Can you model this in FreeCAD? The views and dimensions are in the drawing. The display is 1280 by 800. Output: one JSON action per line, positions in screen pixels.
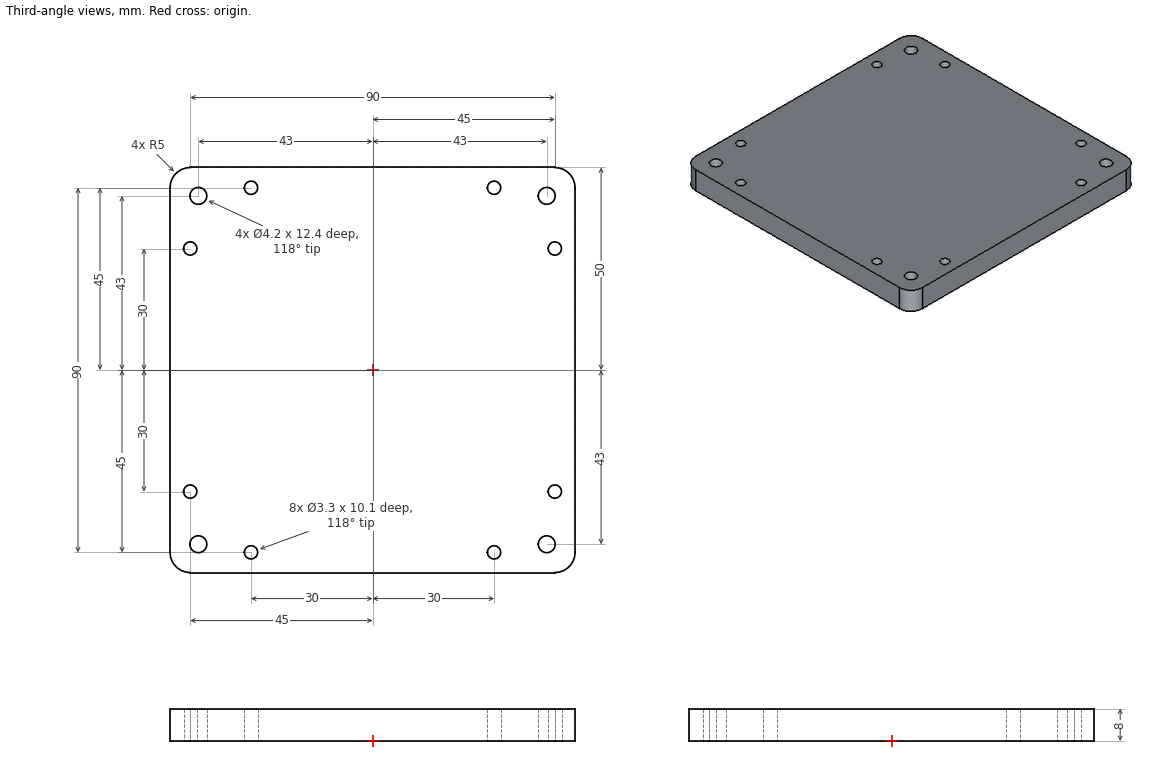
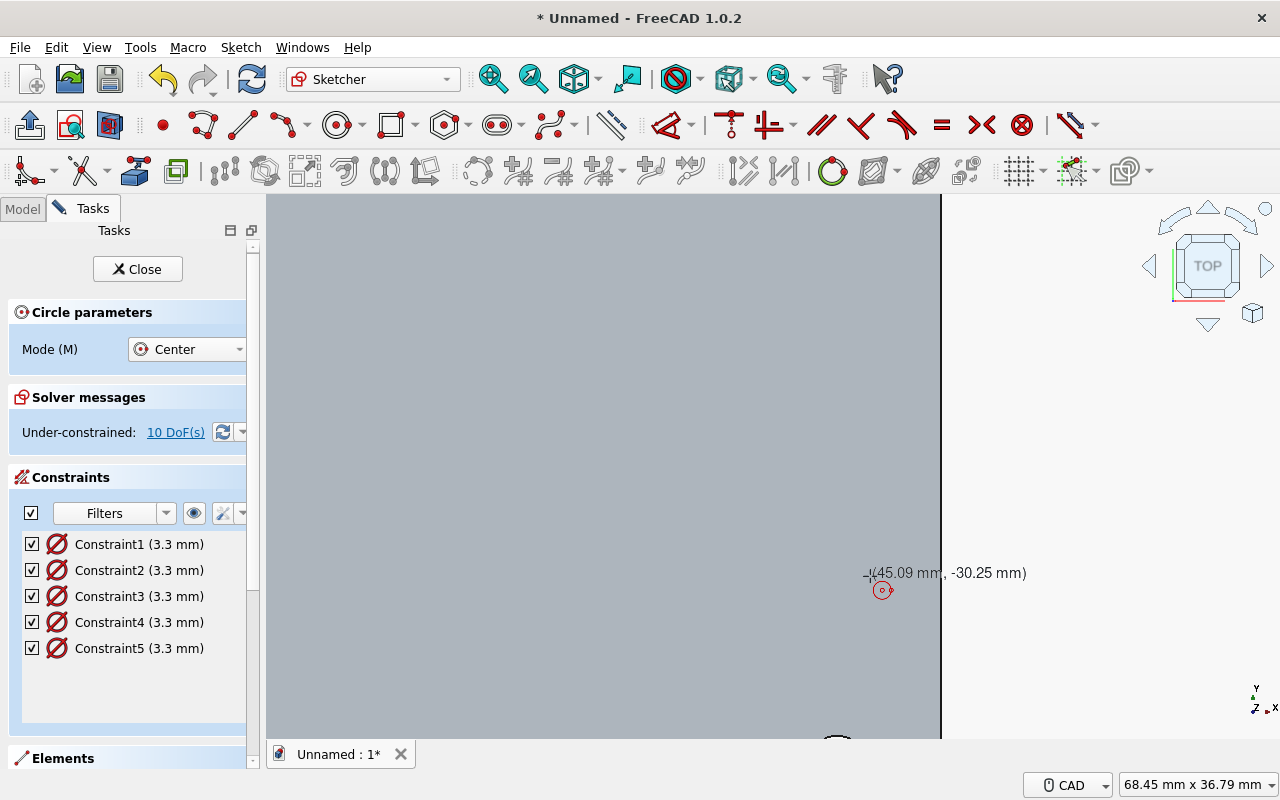
{"action": "scroll", "coordinate": [870, 577], "scroll_direction": "down", "scroll_amount": 7}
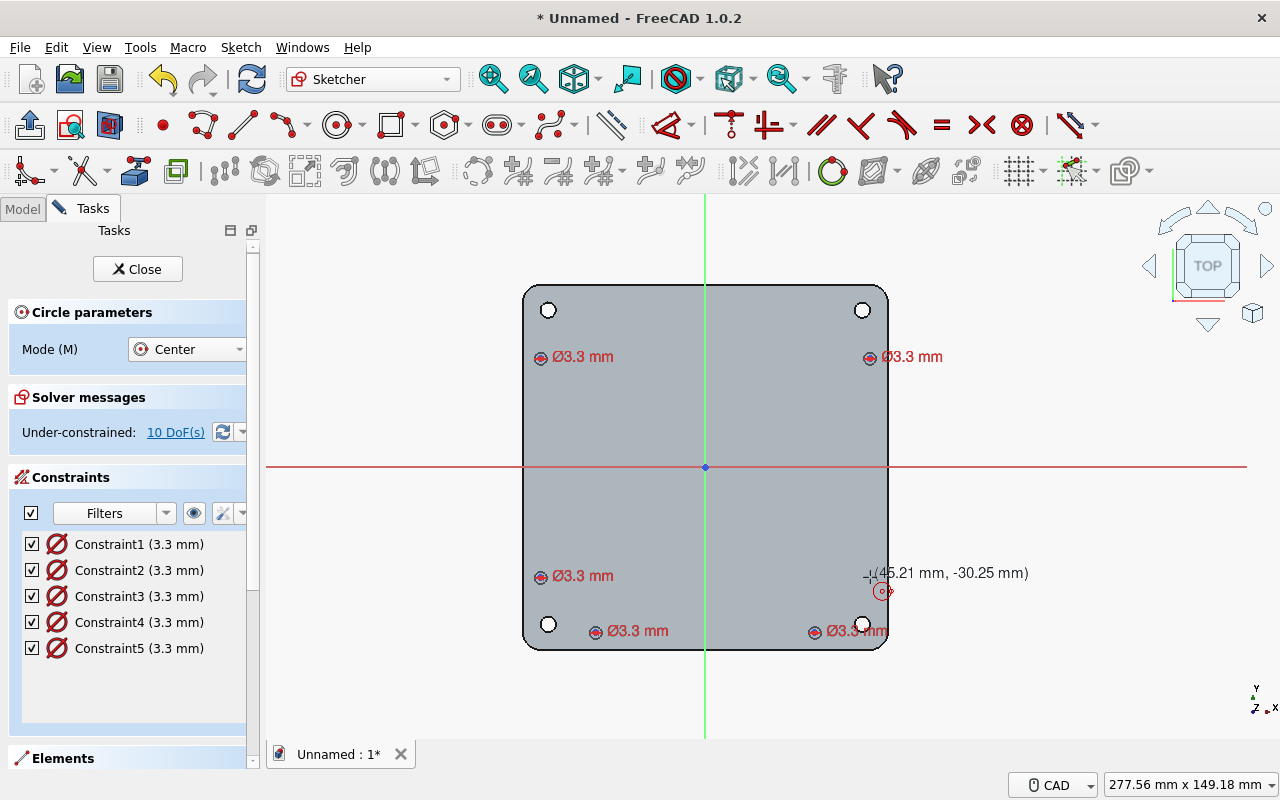
{"action": "left_click", "coordinate": [870, 577]}
{"action": "mouse_move", "coordinate": [874, 573]}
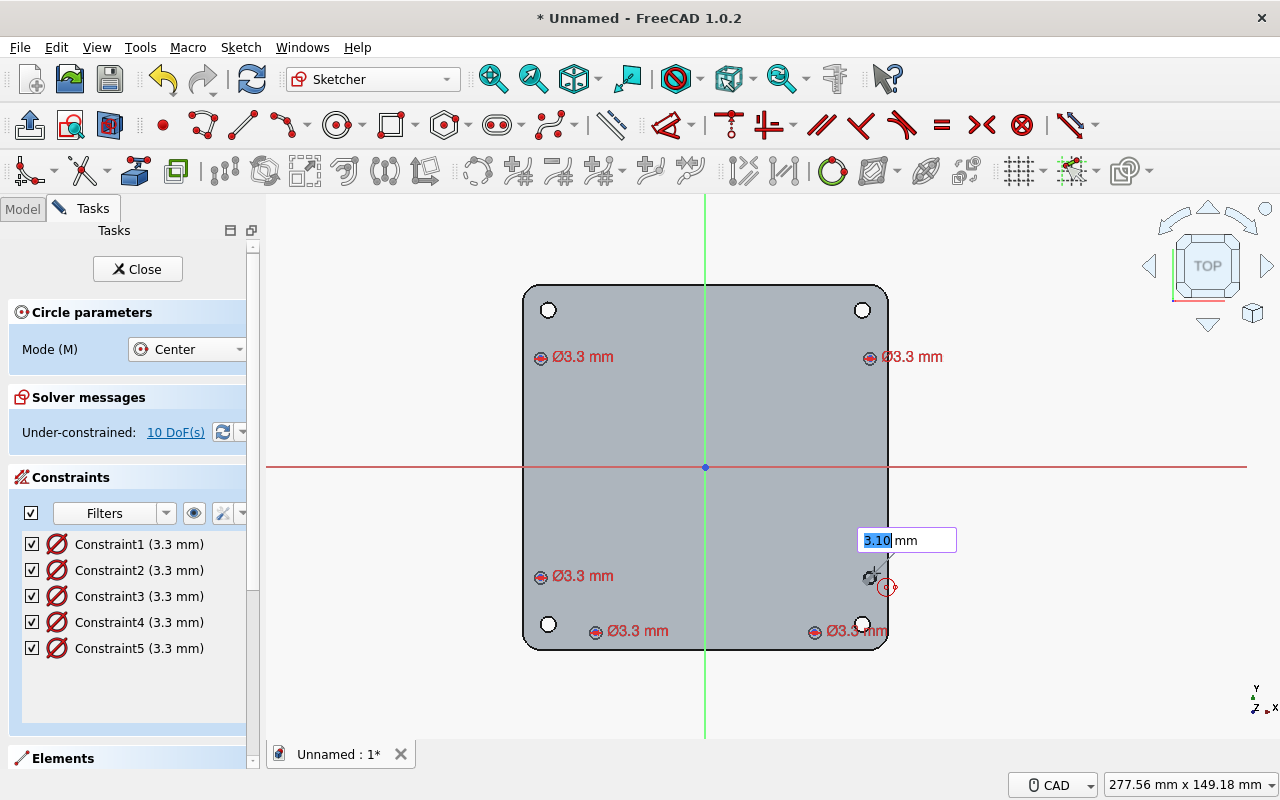
{"action": "type", "text": "3.3"}
{"action": "key", "text": "Return"}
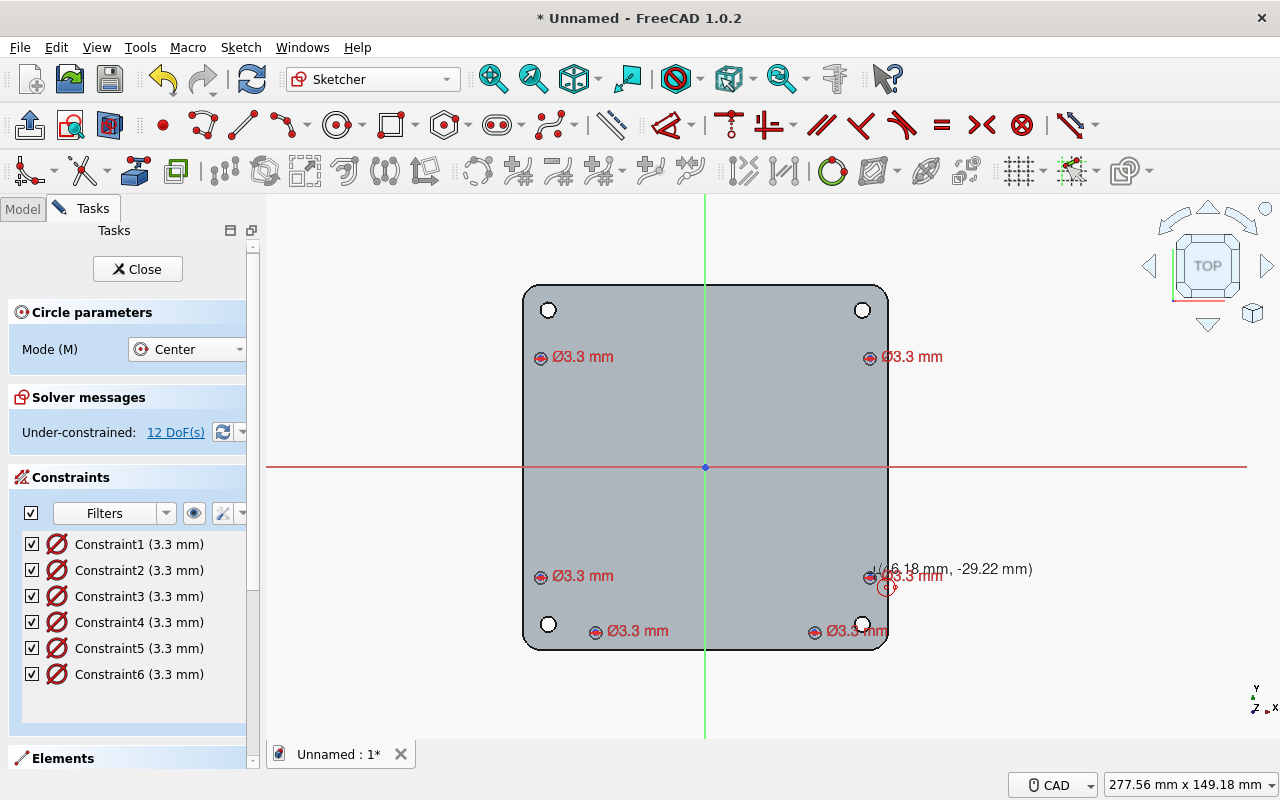
{"action": "scroll", "coordinate": [596, 303], "scroll_direction": "up", "scroll_amount": 7}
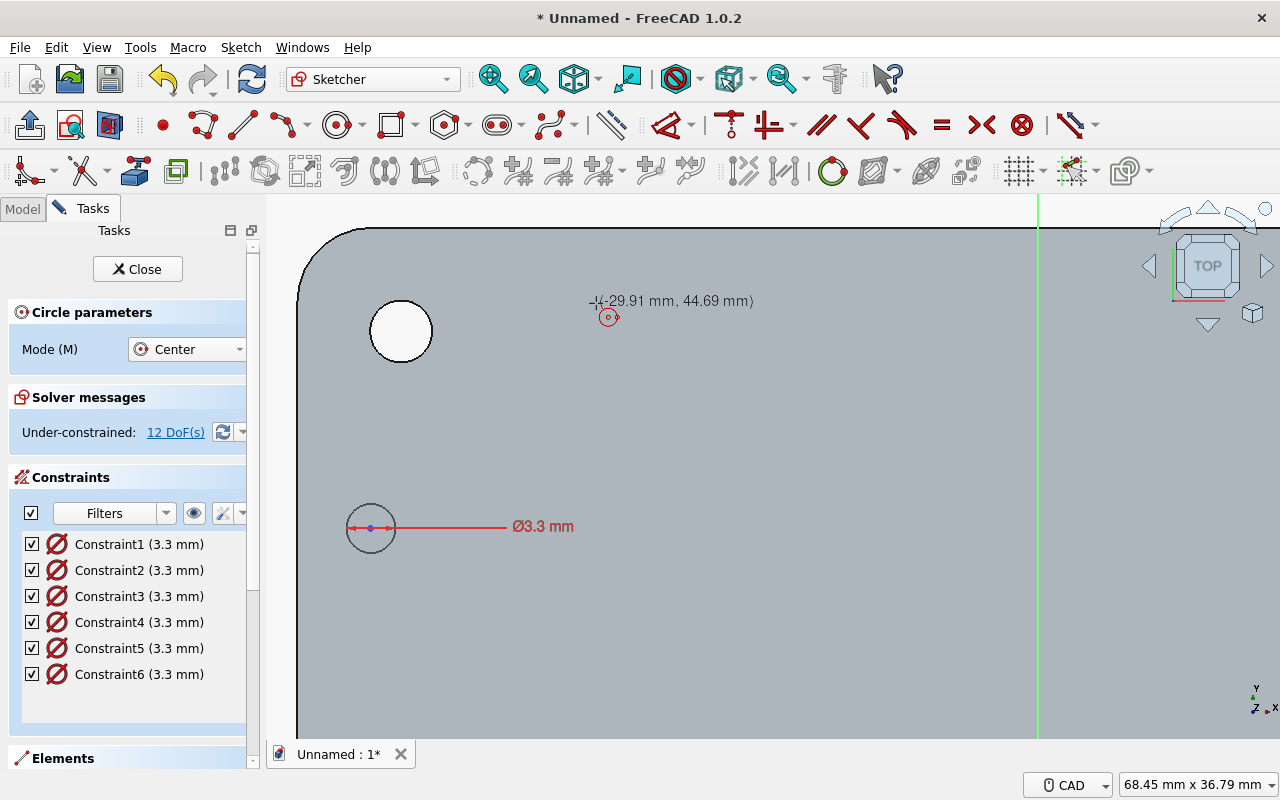
{"action": "scroll", "coordinate": [595, 302], "scroll_direction": "down", "scroll_amount": 7}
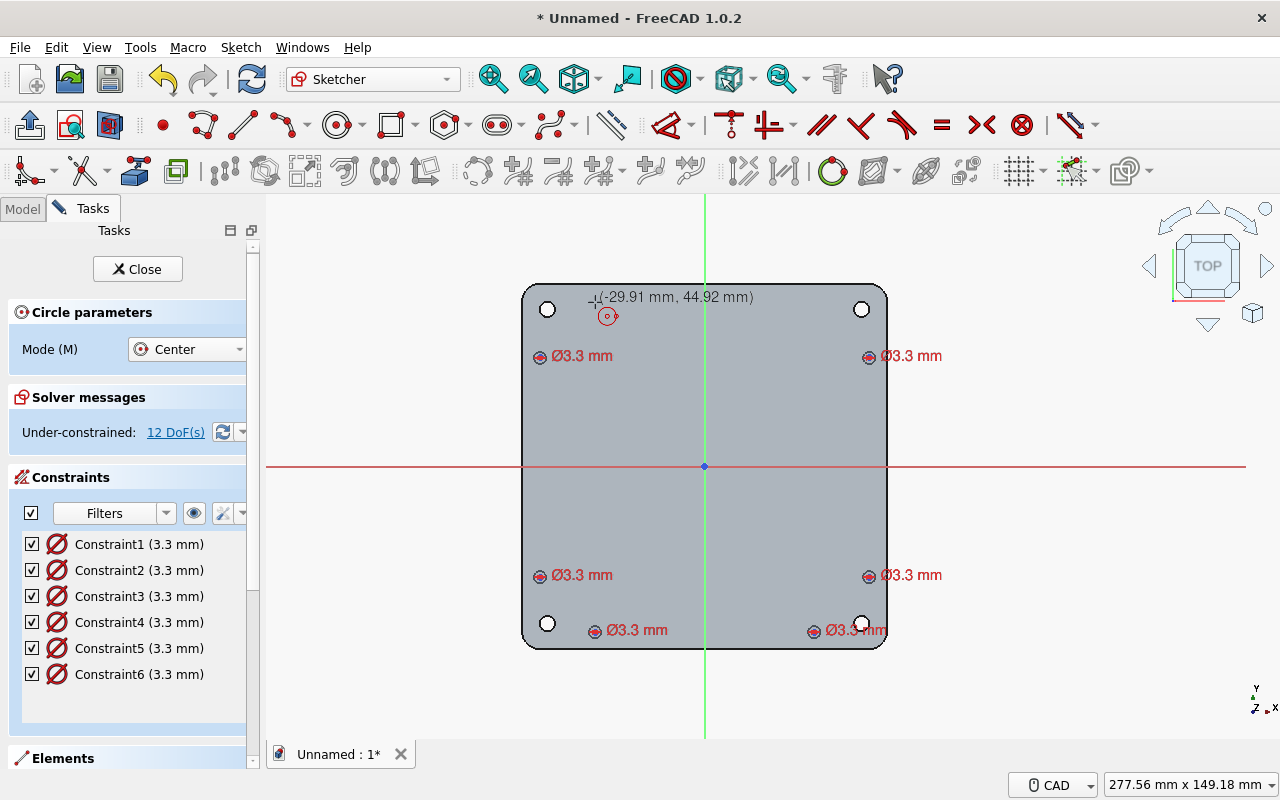
{"action": "left_click", "coordinate": [595, 302]}
{"action": "mouse_move", "coordinate": [599, 298]}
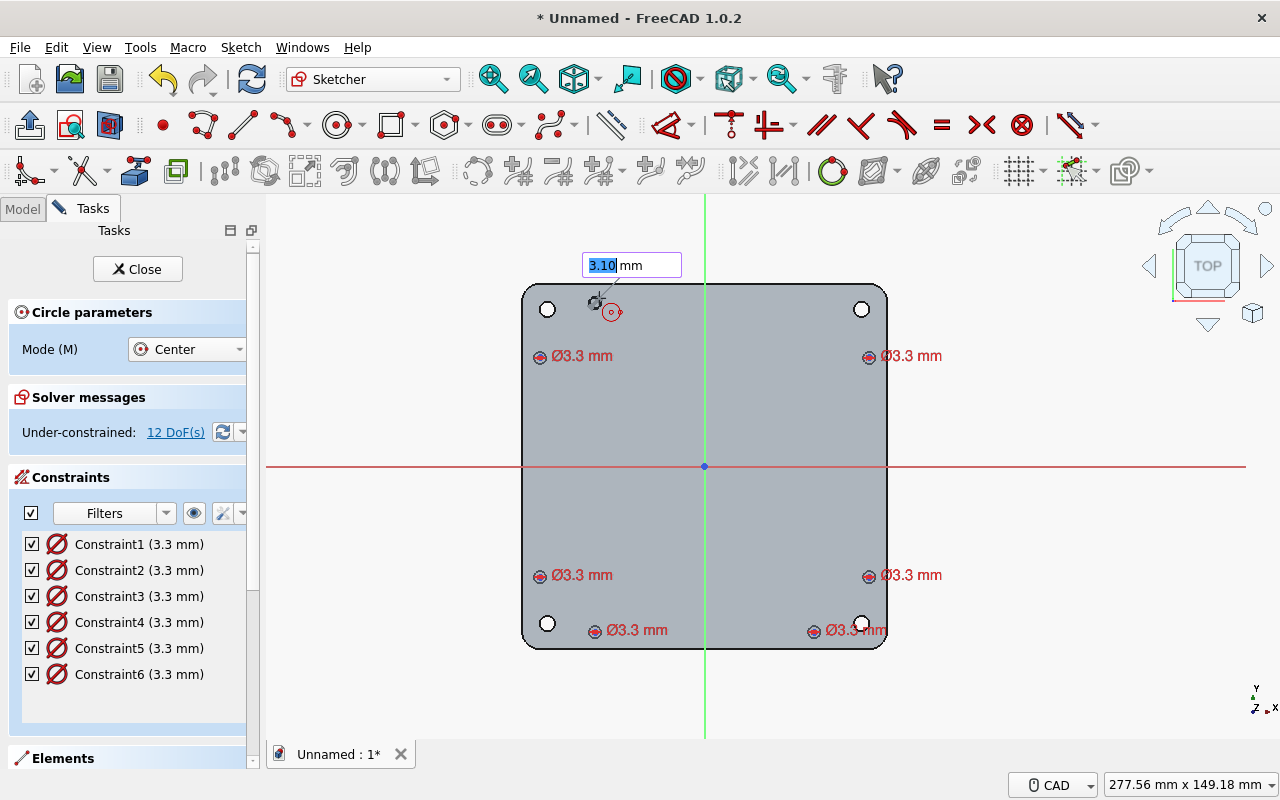
{"action": "type", "text": "3.3"}
{"action": "key", "text": "Return"}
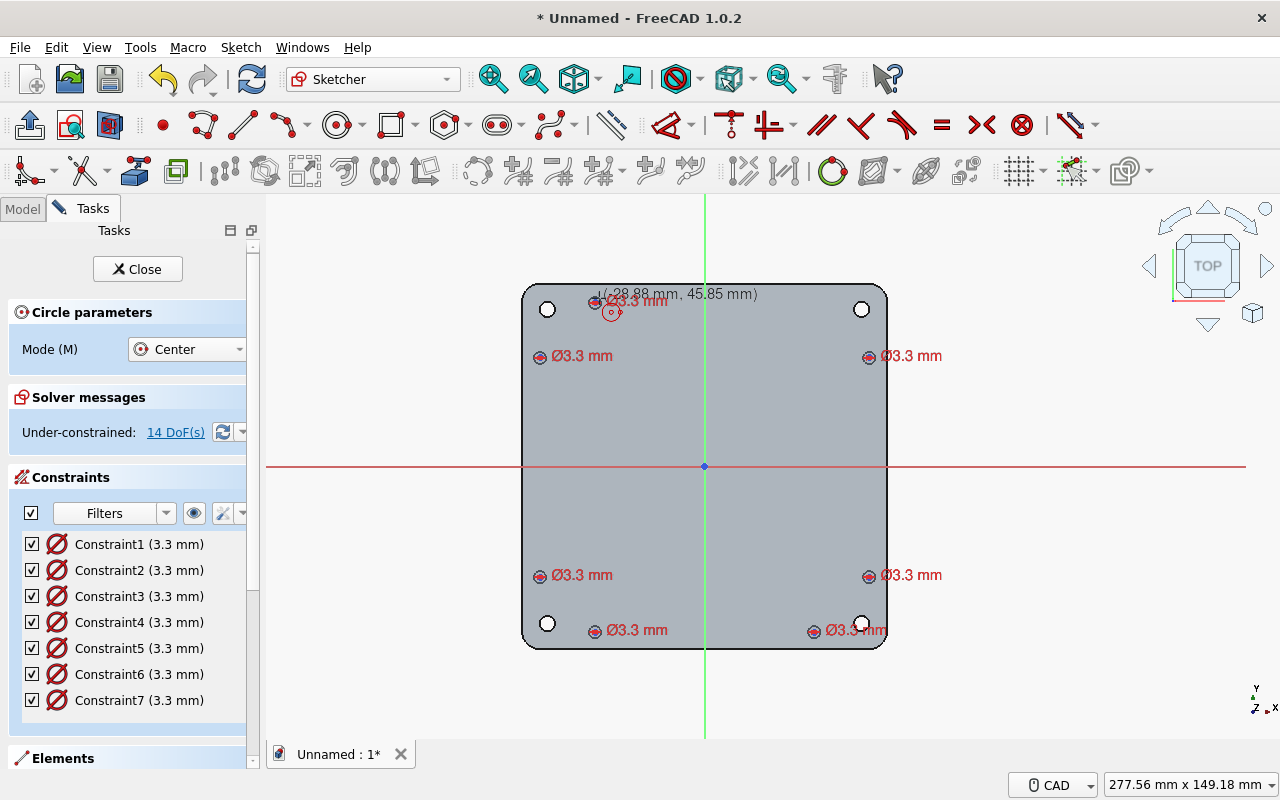
{"action": "scroll", "coordinate": [814, 302], "scroll_direction": "up", "scroll_amount": 7}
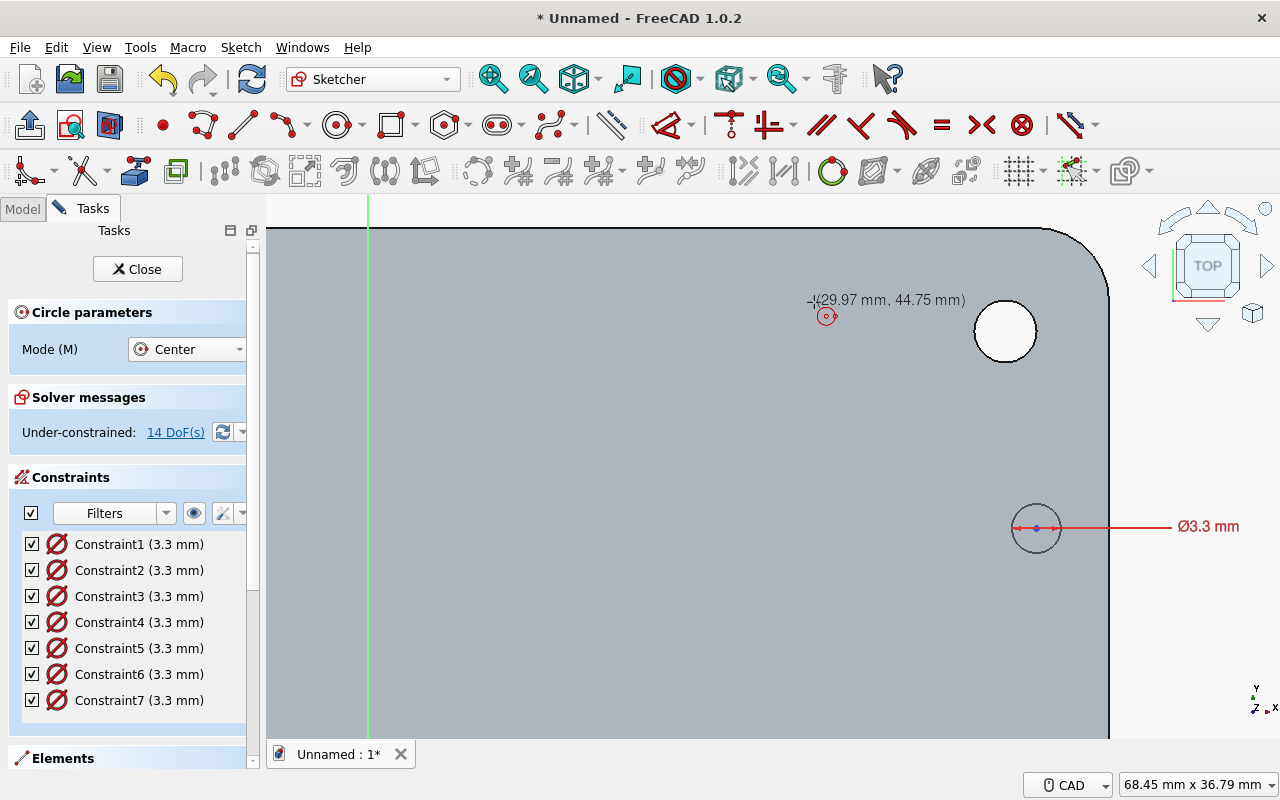
{"action": "scroll", "coordinate": [815, 302], "scroll_direction": "down", "scroll_amount": 7}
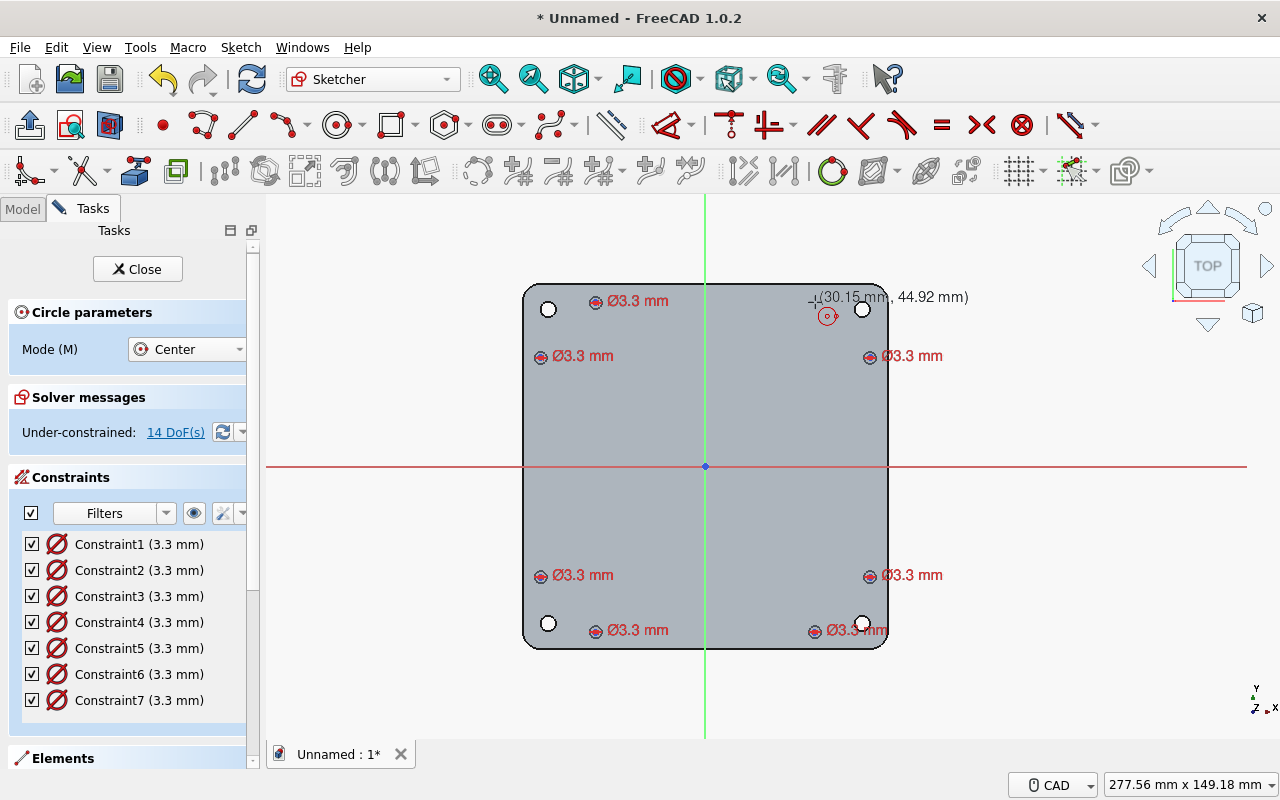
{"action": "left_click", "coordinate": [815, 302]}
{"action": "mouse_move", "coordinate": [819, 298]}